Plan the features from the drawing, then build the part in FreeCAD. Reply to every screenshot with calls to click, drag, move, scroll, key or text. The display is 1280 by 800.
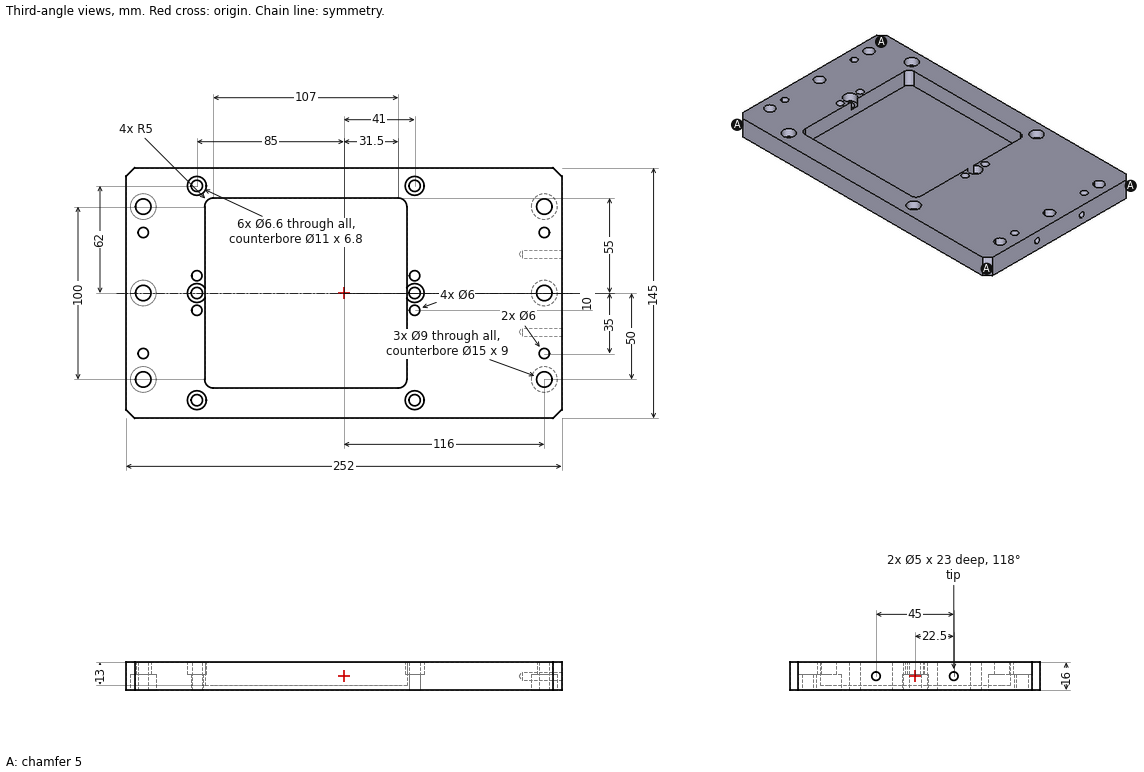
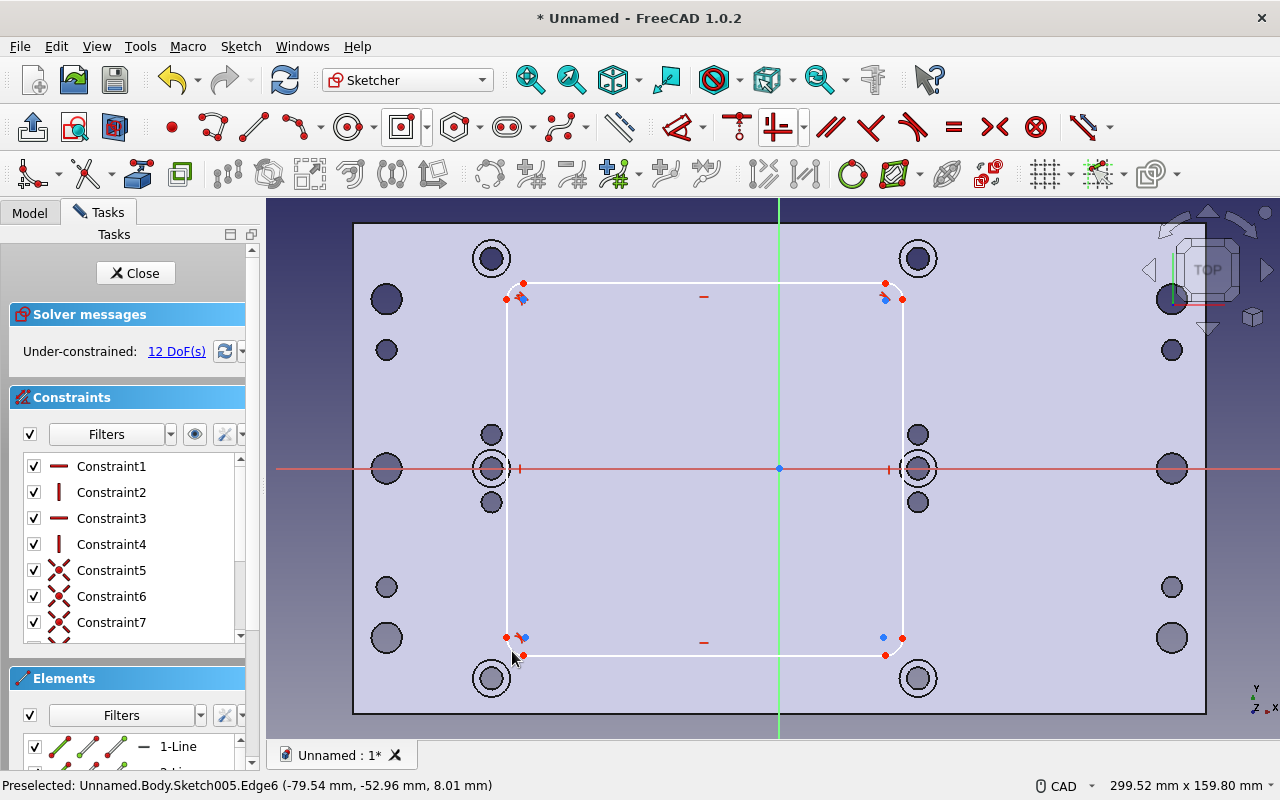
click(633, 656)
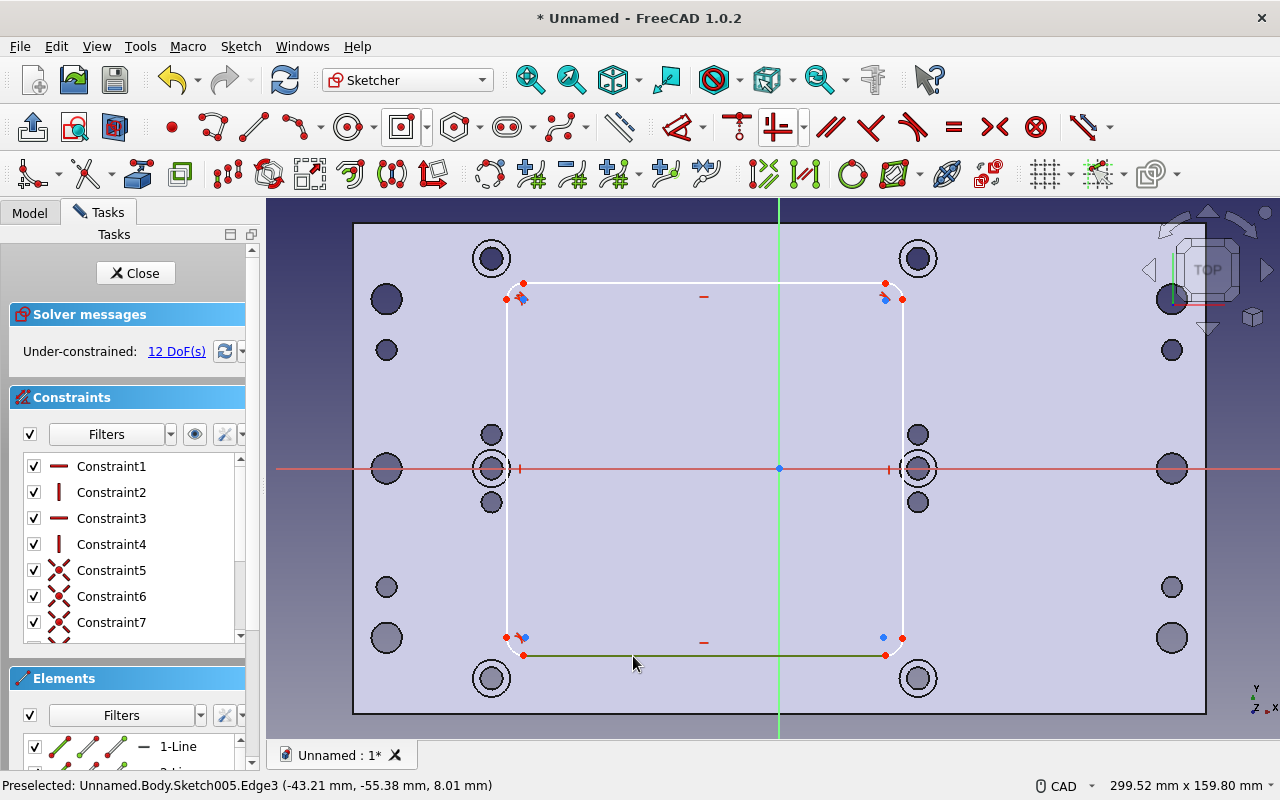
click(512, 650)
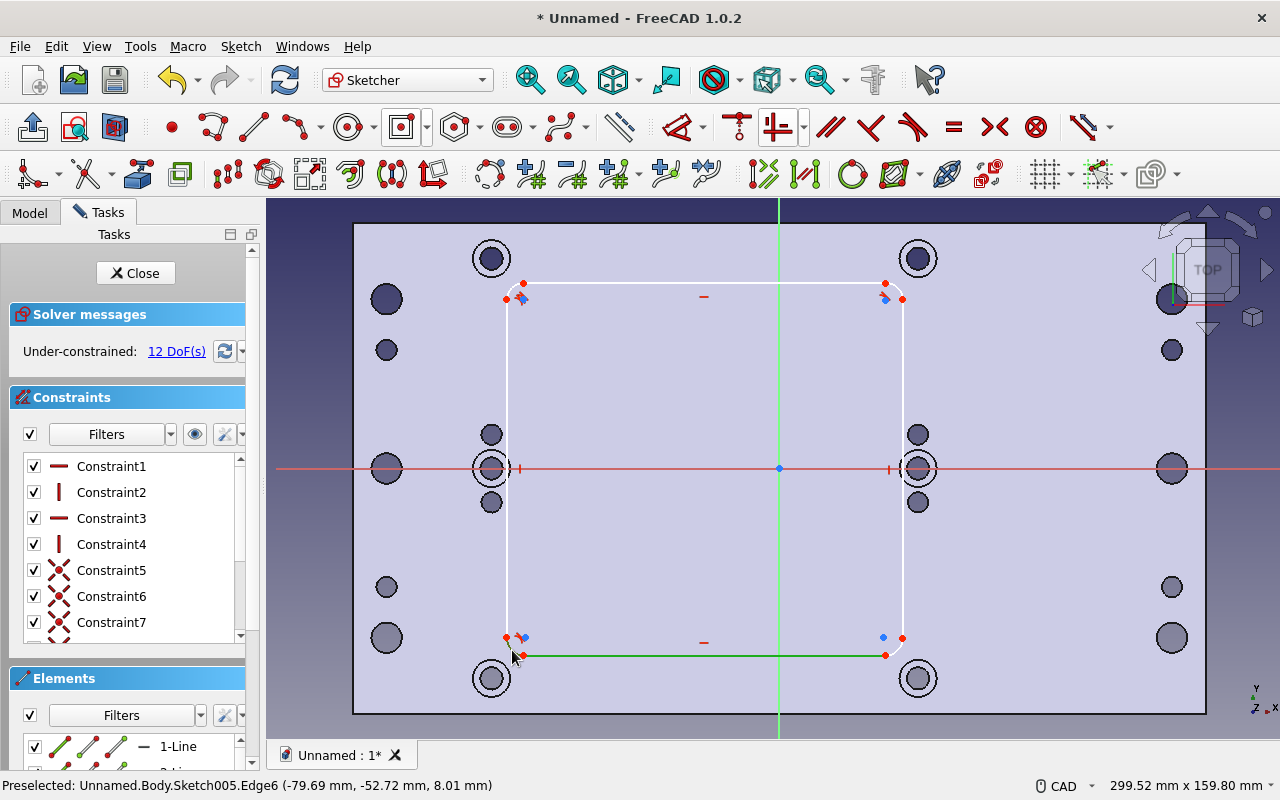
key(t)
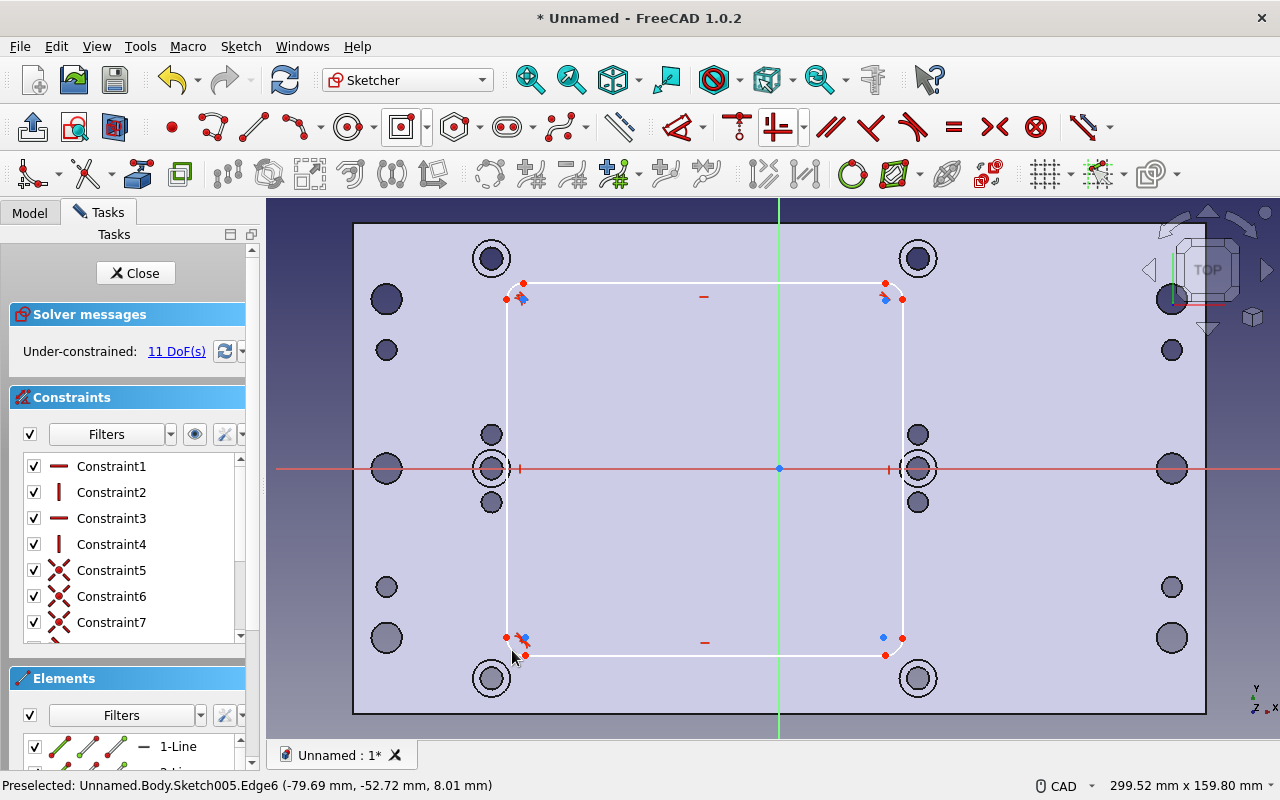
click(634, 656)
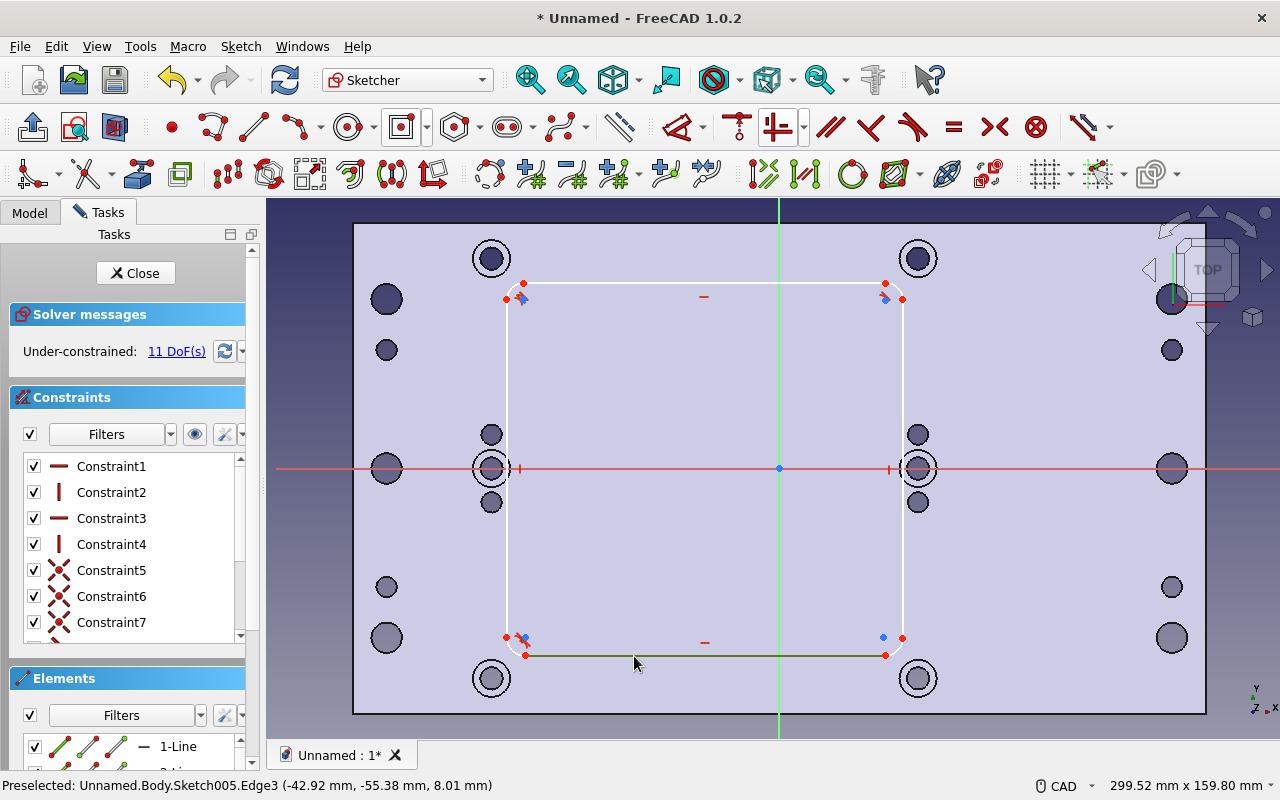
click(897, 651)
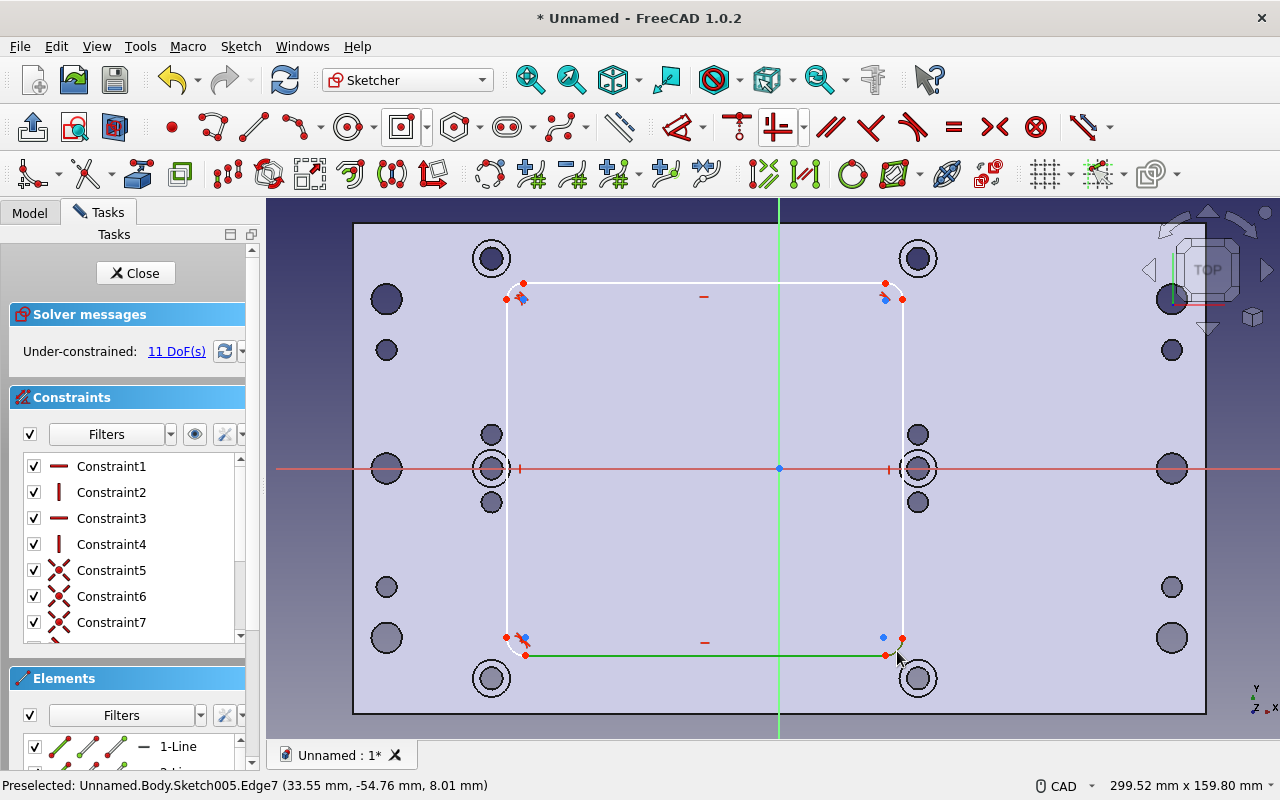
key(t)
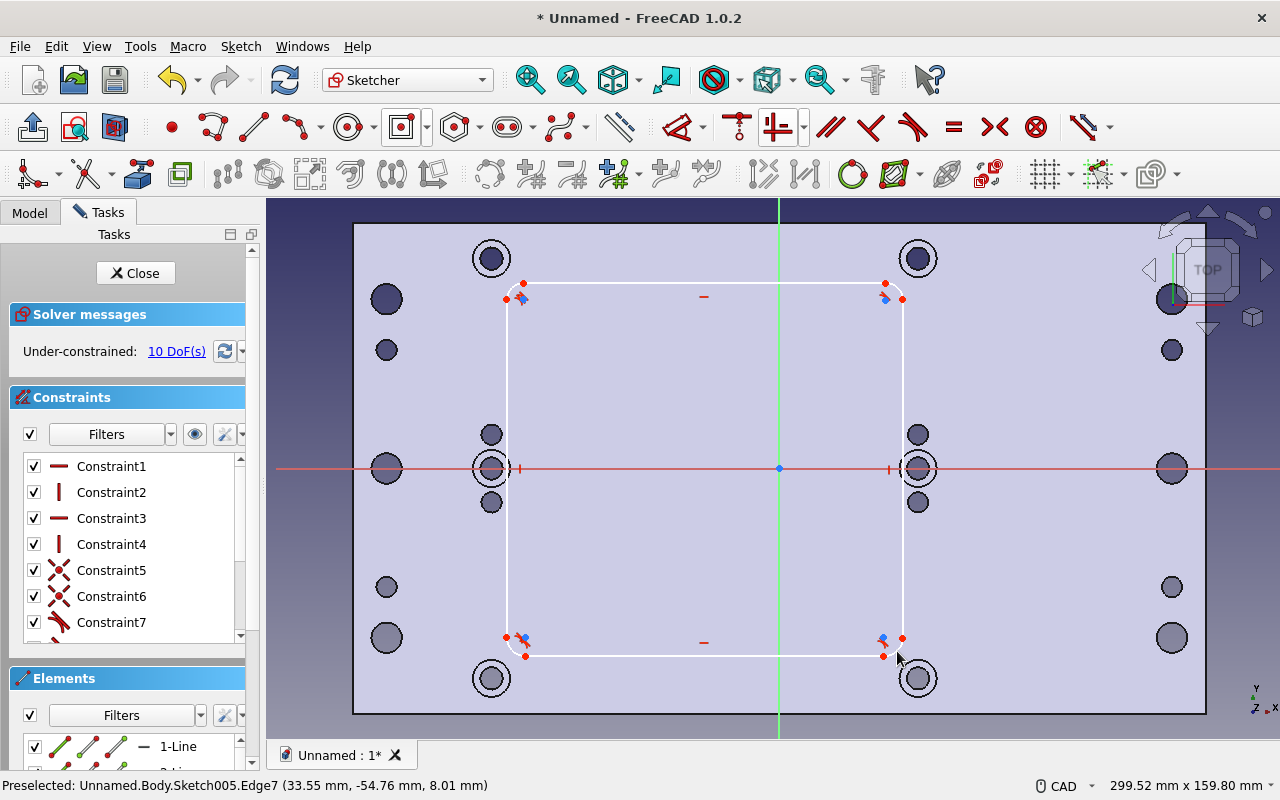
click(903, 537)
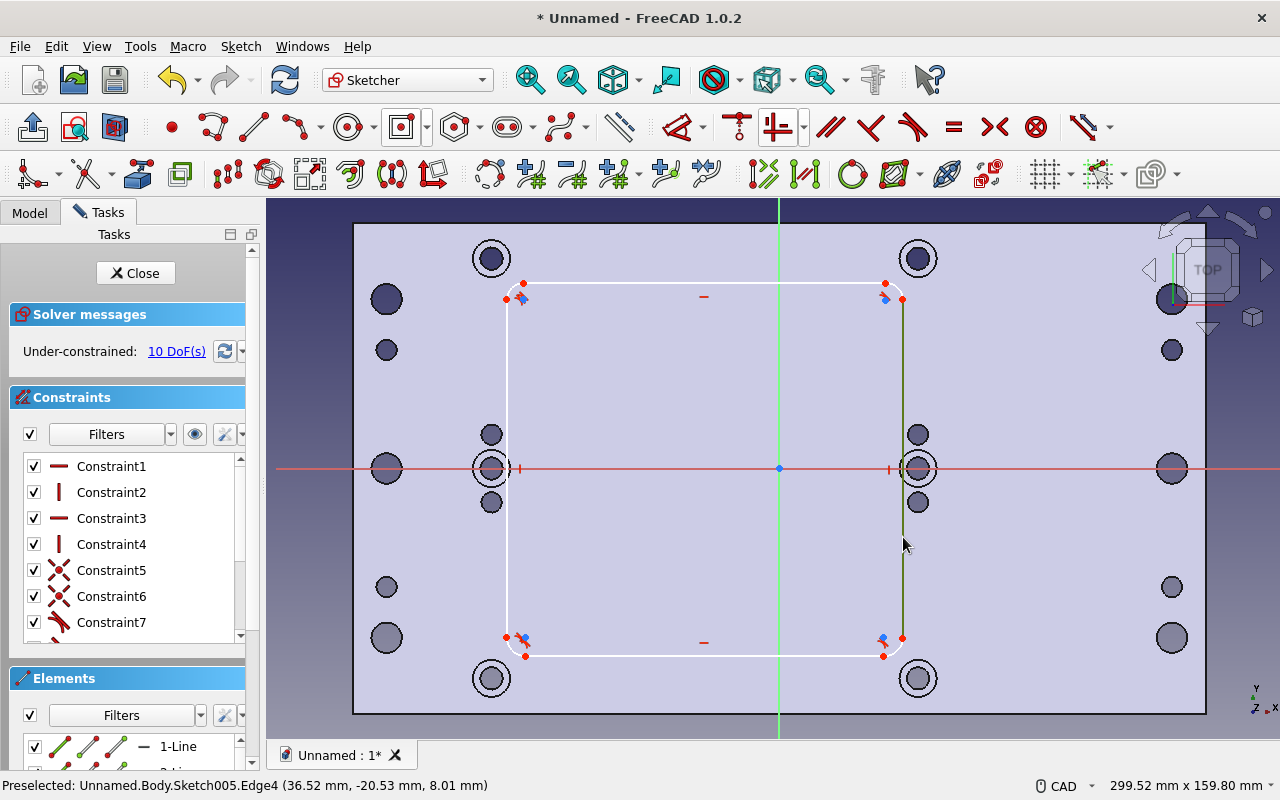
click(897, 651)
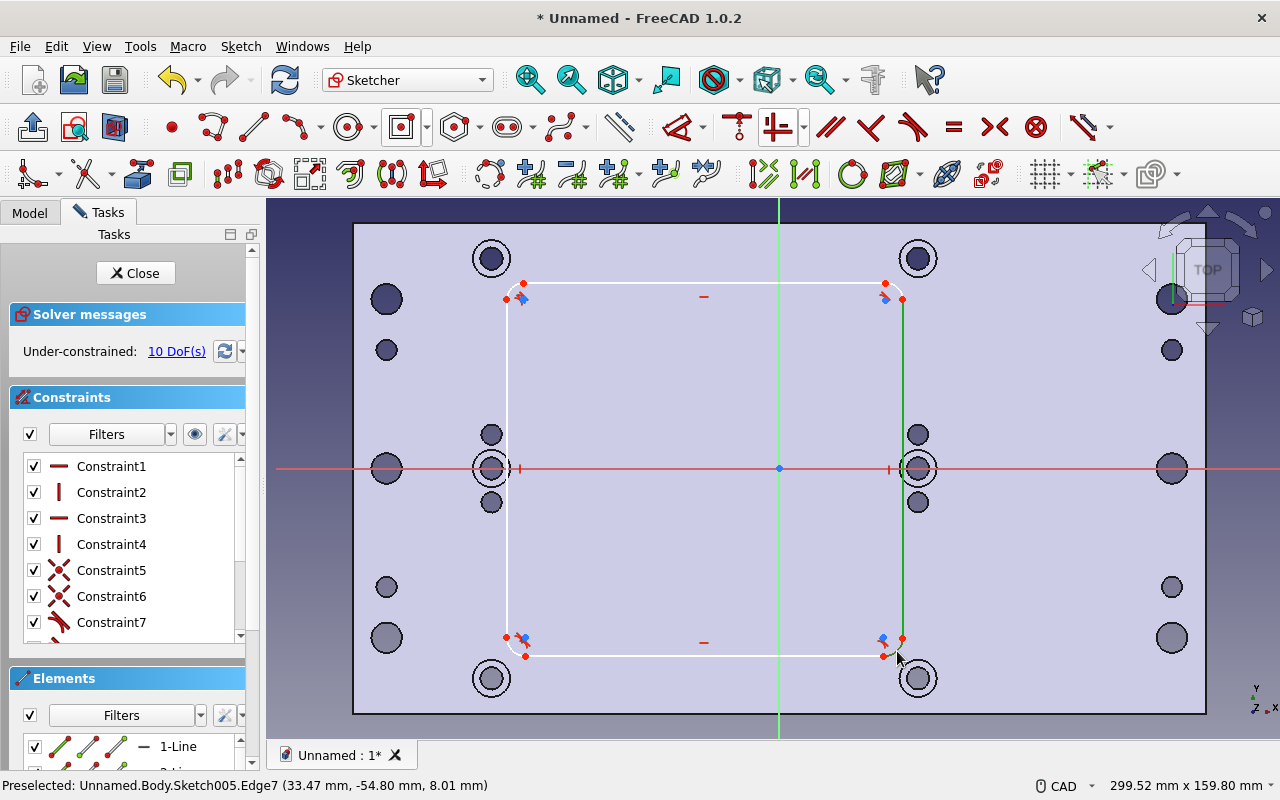
key(t)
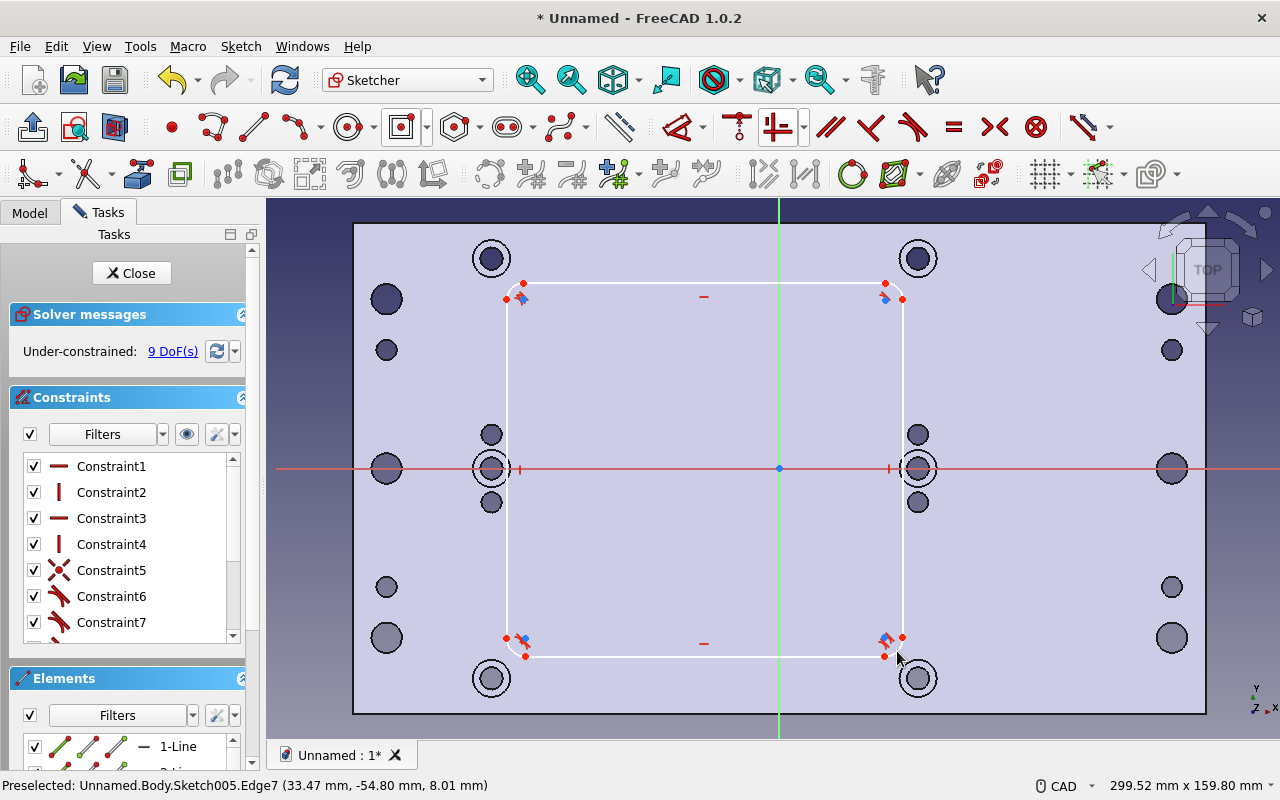
click(903, 536)